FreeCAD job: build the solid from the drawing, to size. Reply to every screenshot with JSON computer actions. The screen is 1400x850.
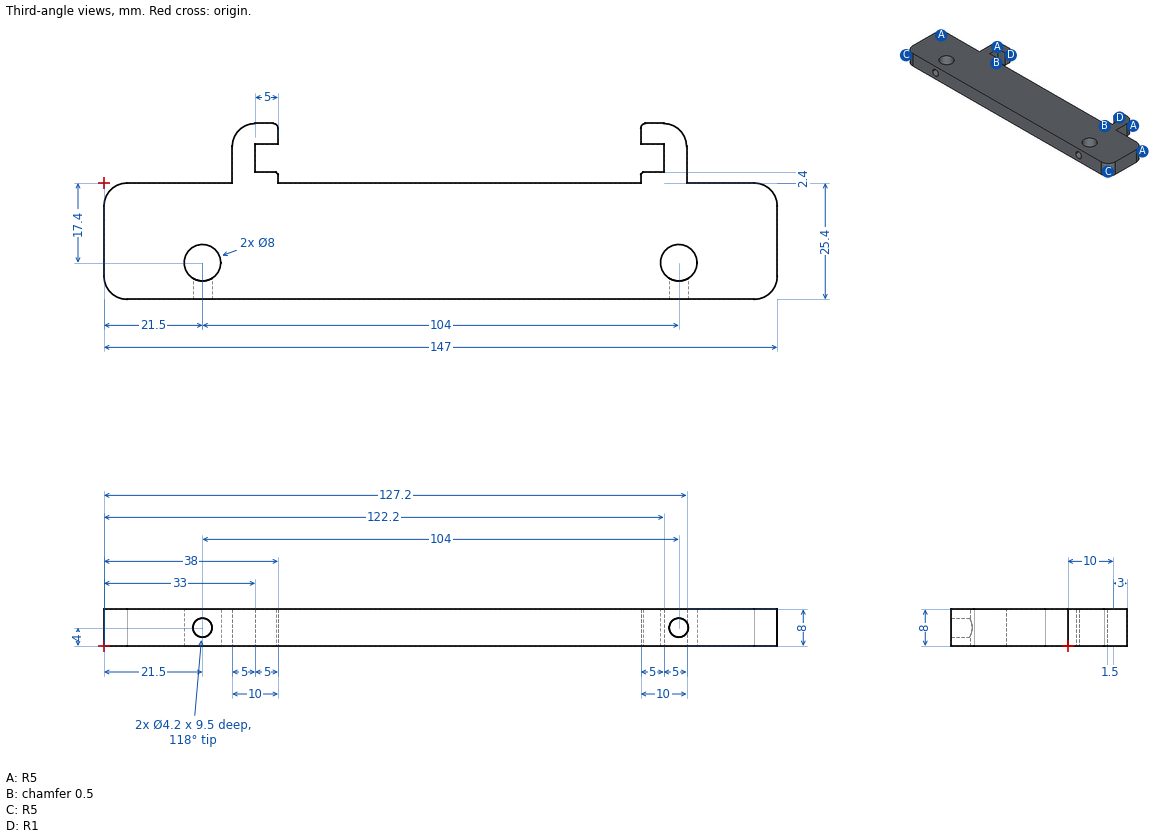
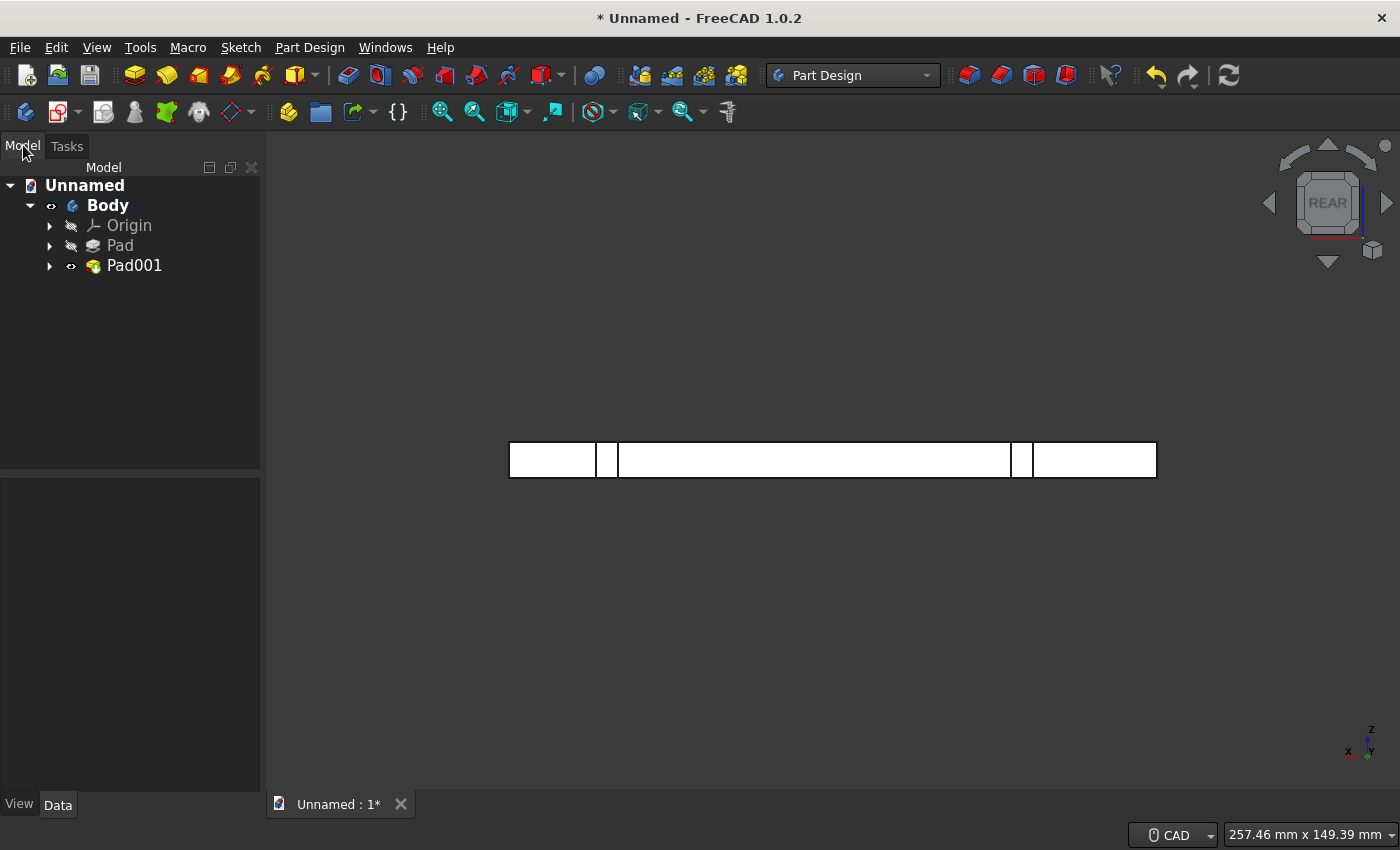
{"action": "left_click", "coordinate": [50, 226]}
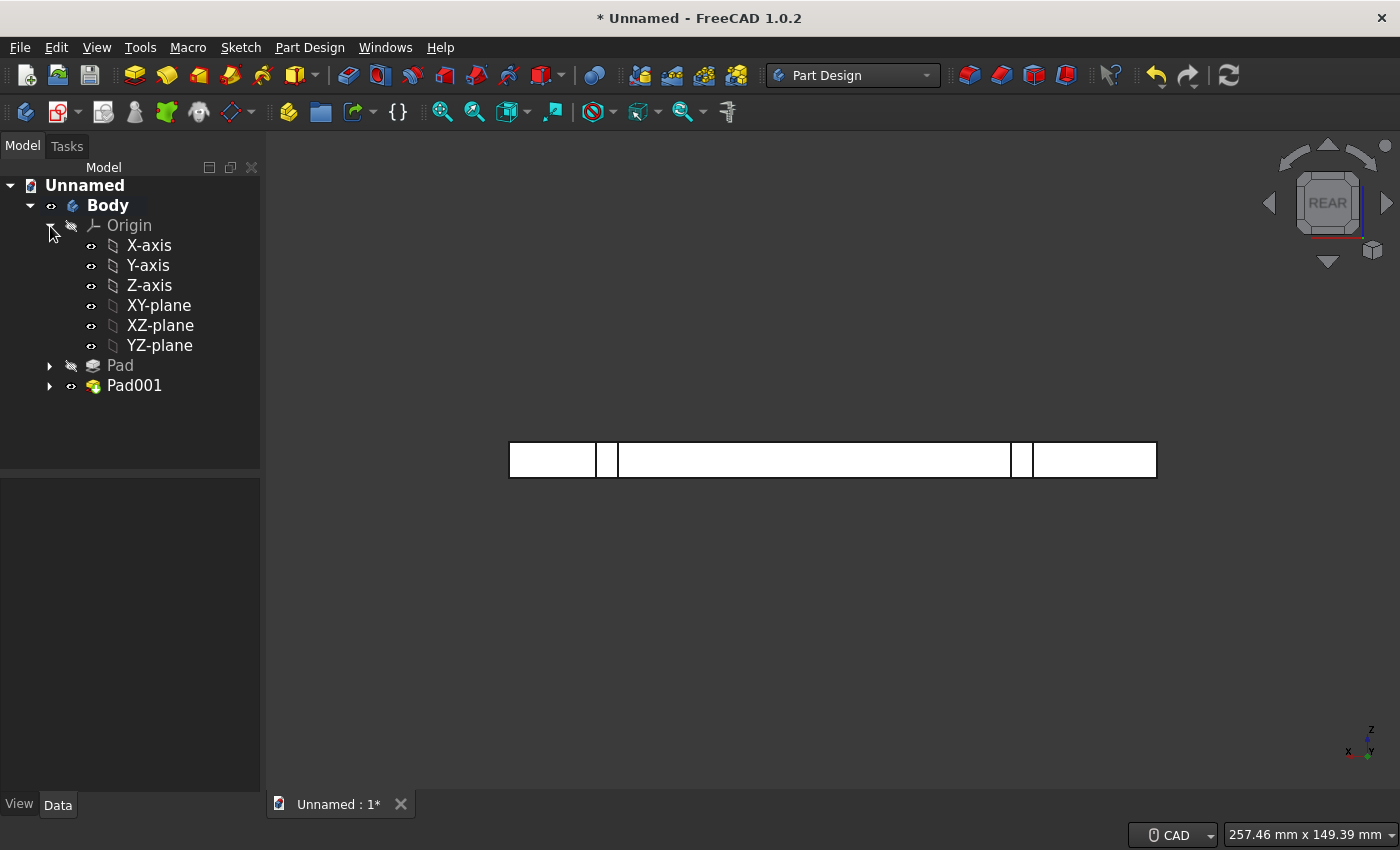
{"action": "left_click", "coordinate": [136, 346]}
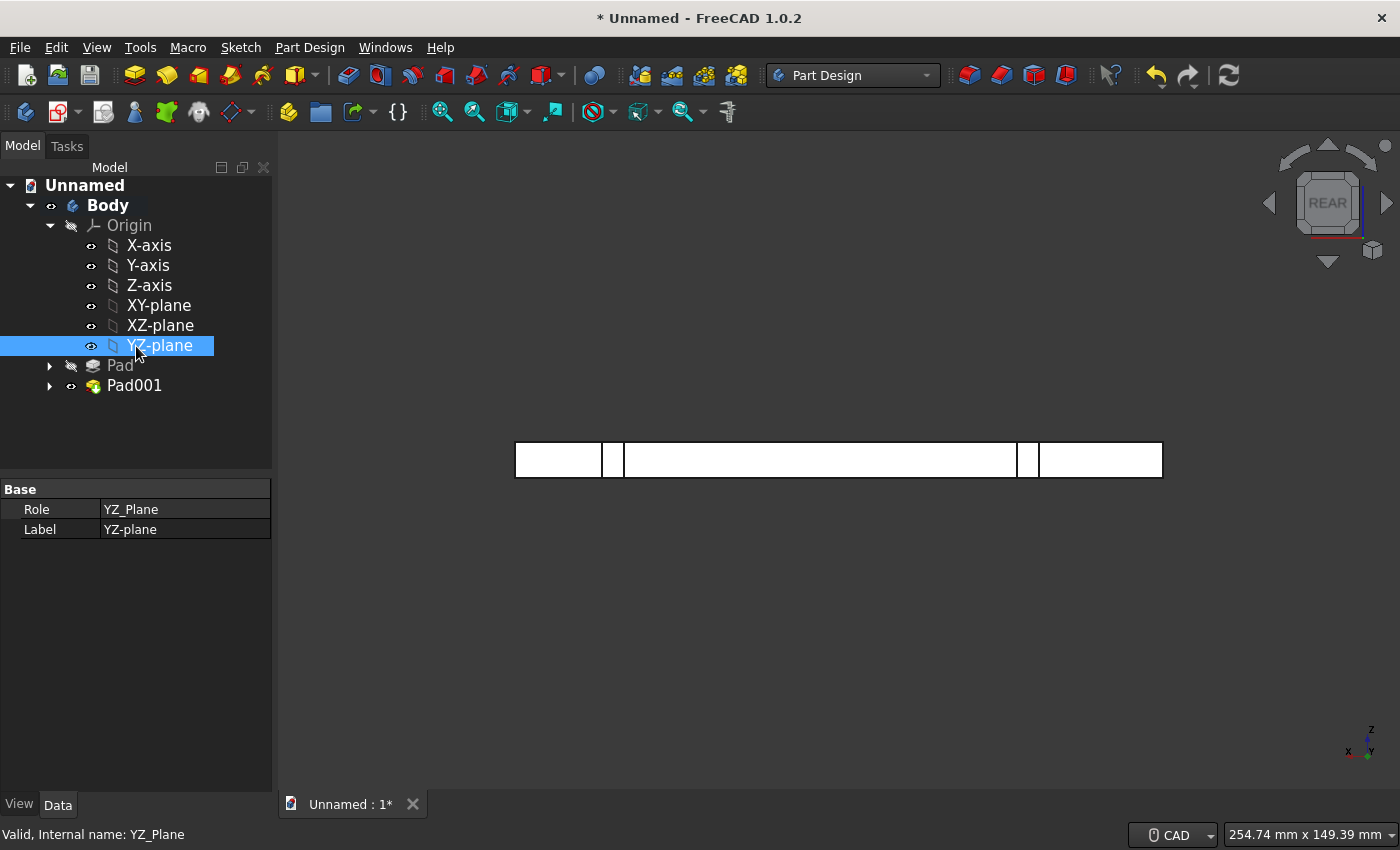
{"action": "left_click", "coordinate": [232, 112]}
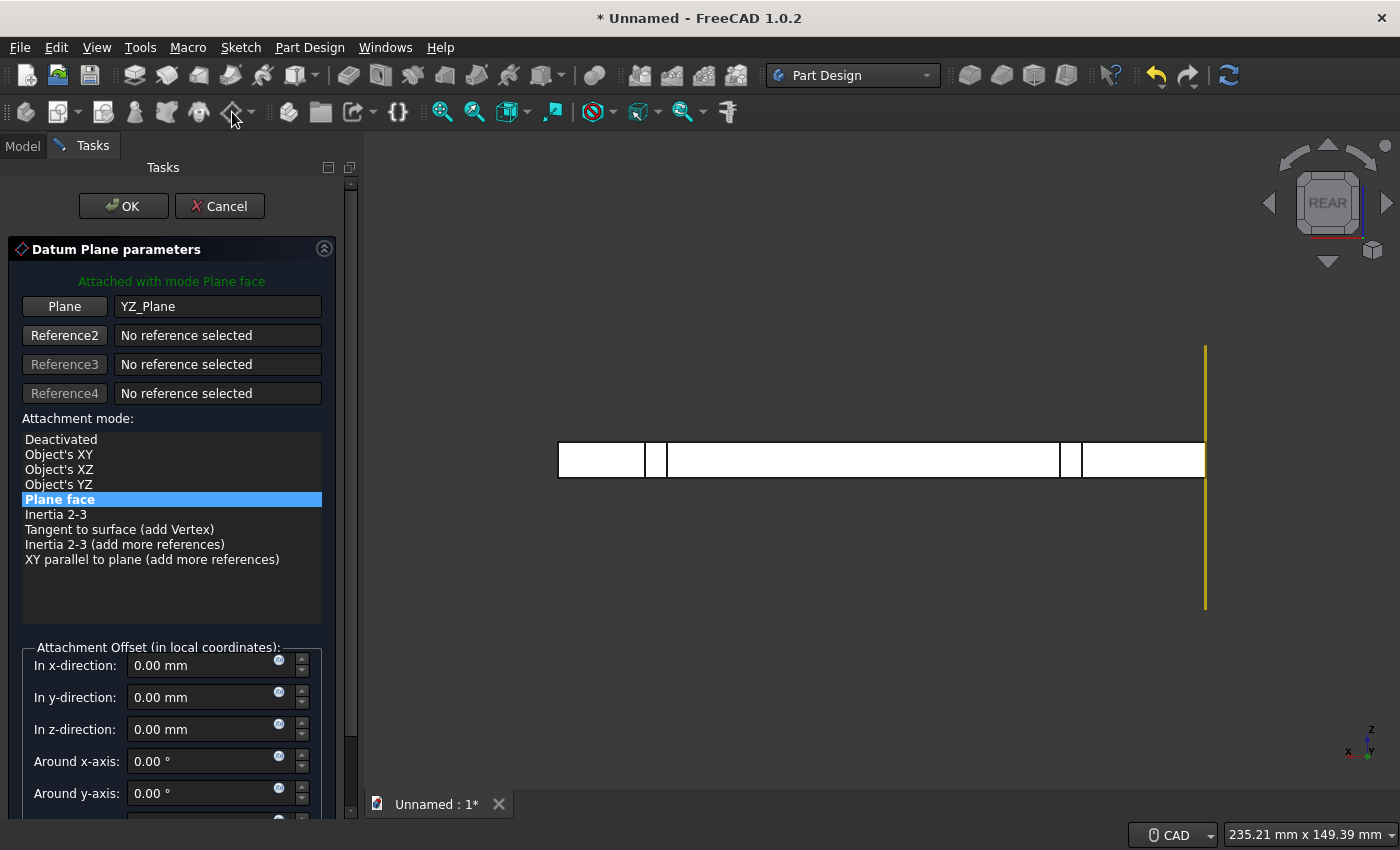
{"action": "triple_click", "coordinate": [210, 729]}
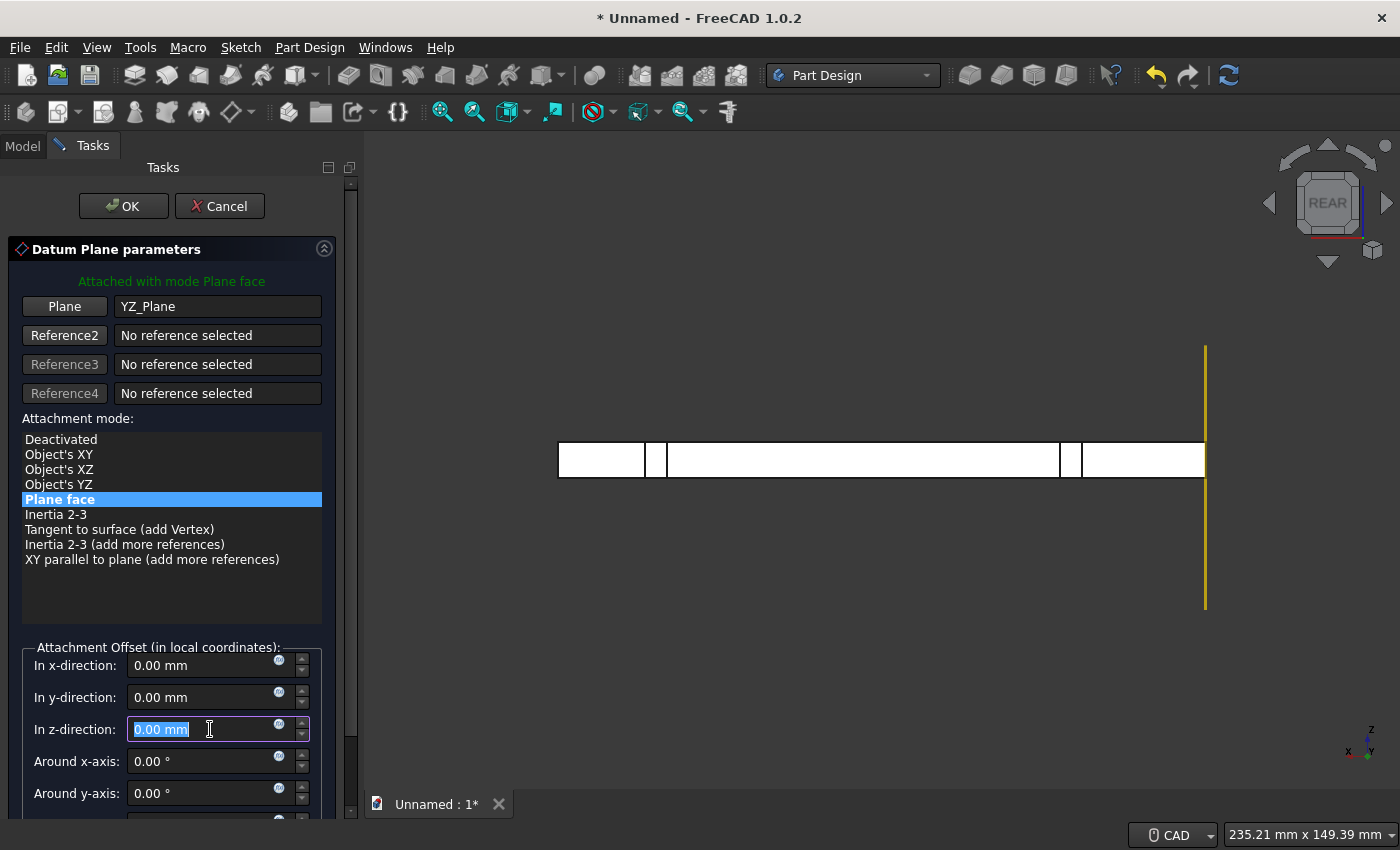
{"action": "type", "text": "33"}
{"action": "key", "text": "Tab"}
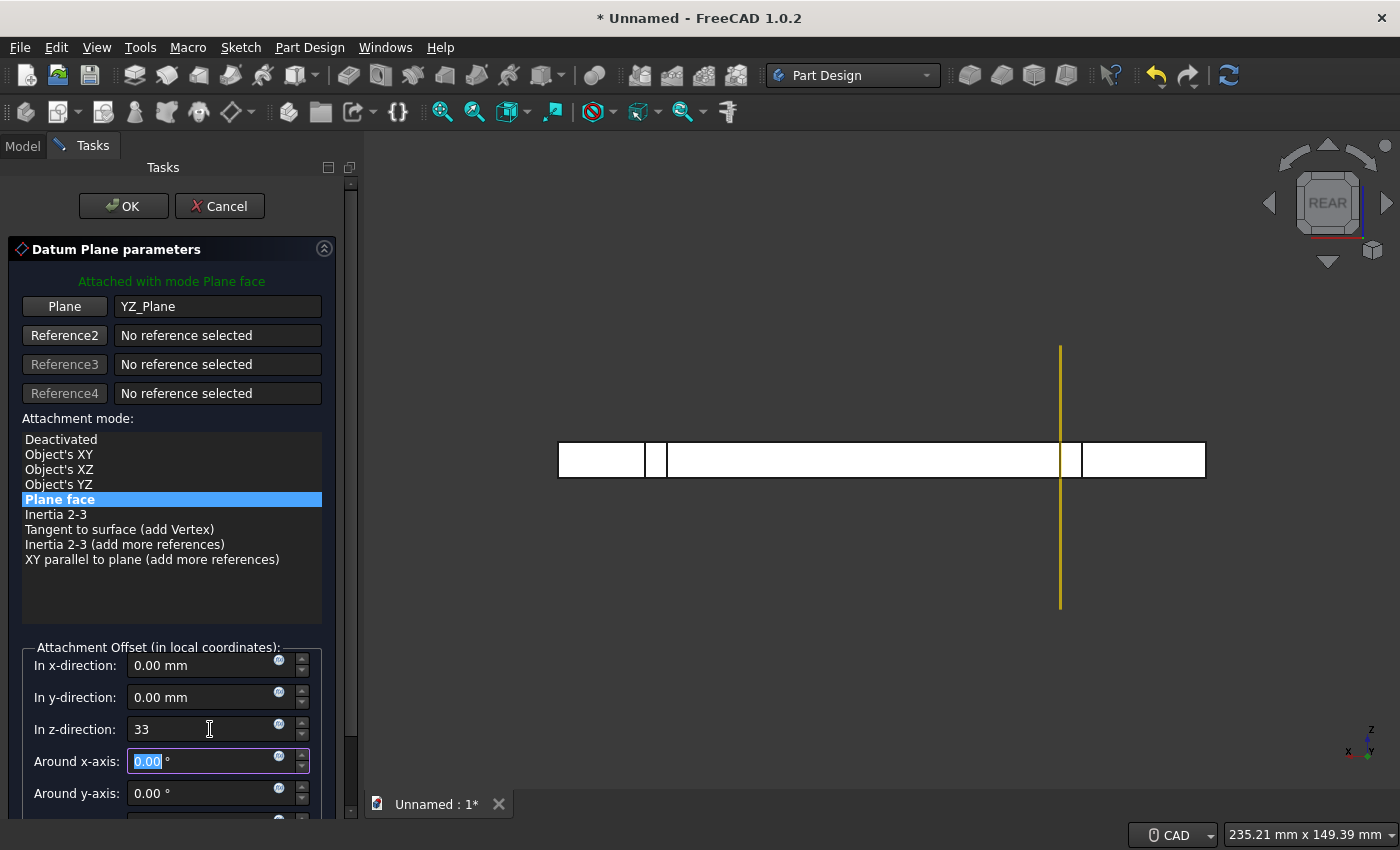
{"action": "left_click", "coordinate": [124, 206]}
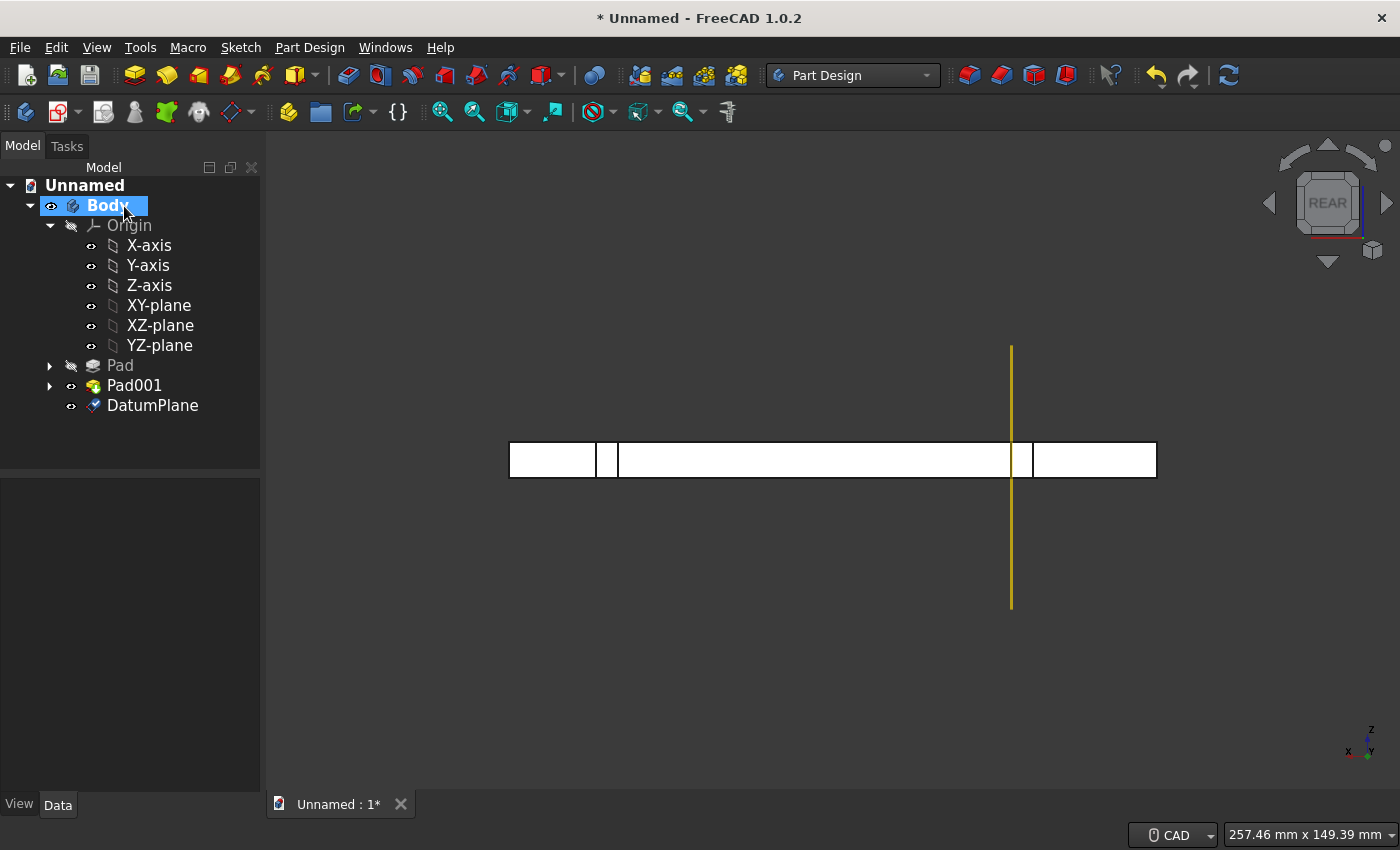
{"action": "left_click", "coordinate": [116, 406]}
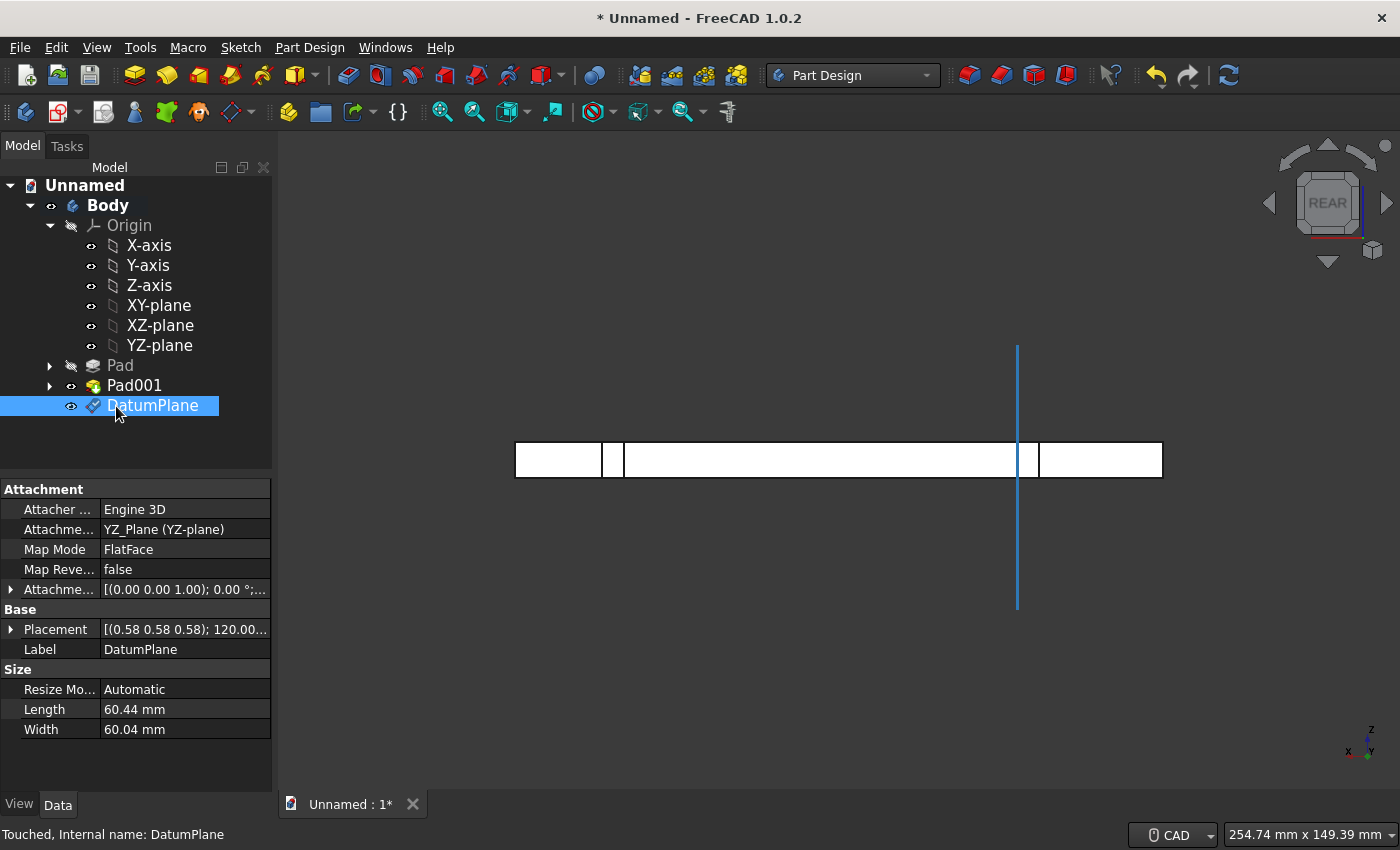
{"action": "left_click", "coordinate": [58, 112]}